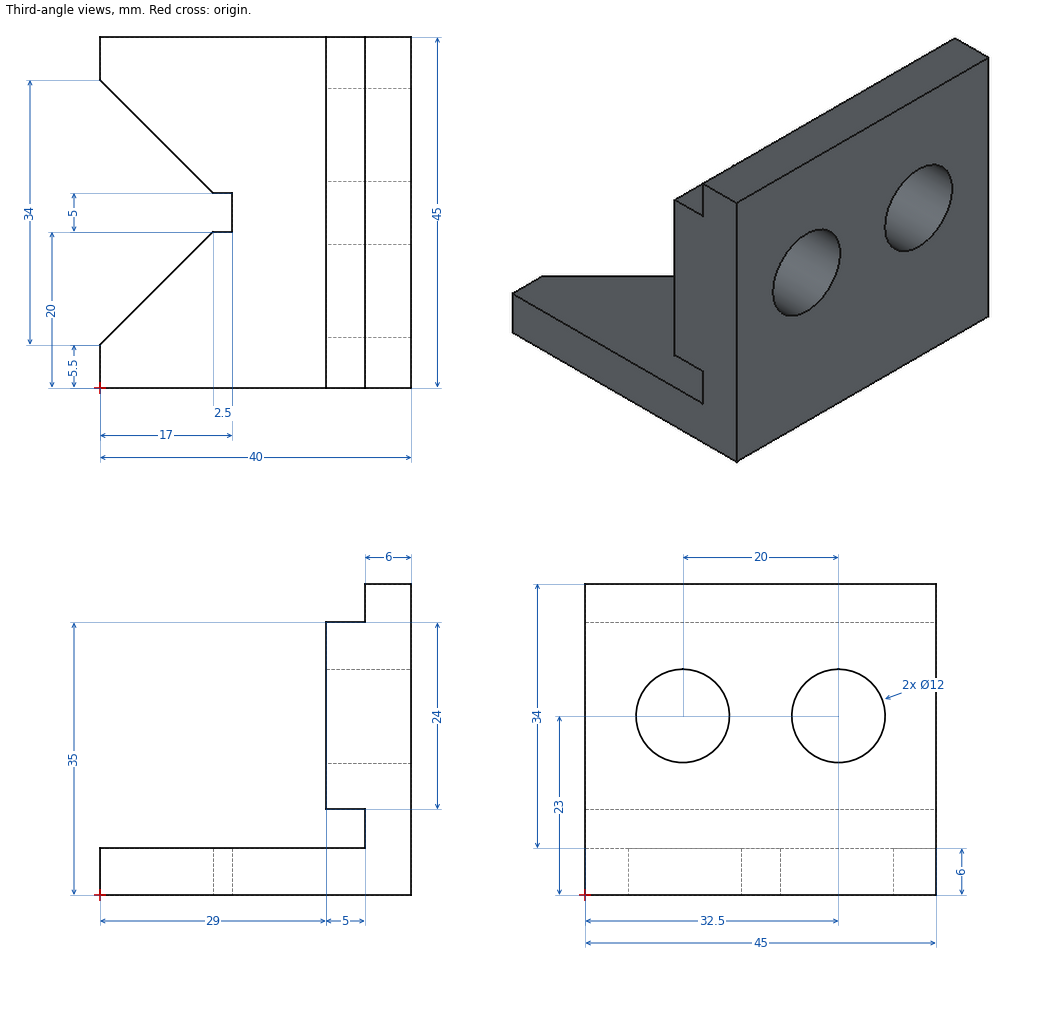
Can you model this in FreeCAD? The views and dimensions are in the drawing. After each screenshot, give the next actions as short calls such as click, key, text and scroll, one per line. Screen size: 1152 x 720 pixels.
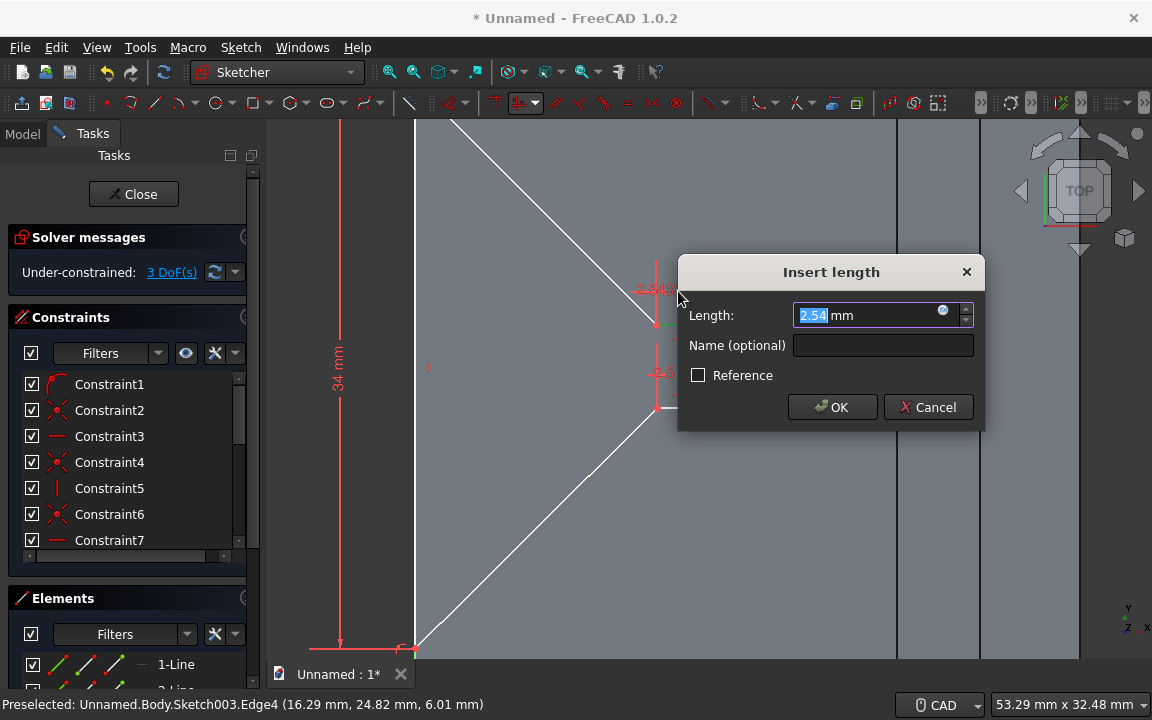
text(2.5)
key(Return)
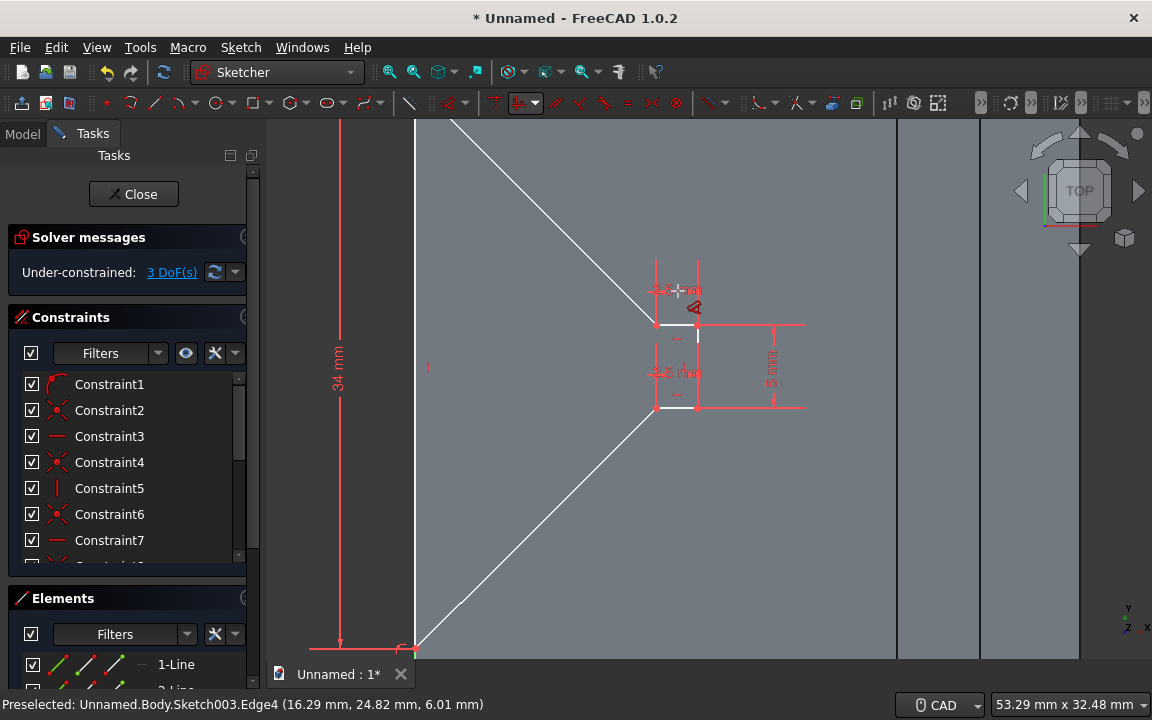
click(656, 408)
click(381, 520)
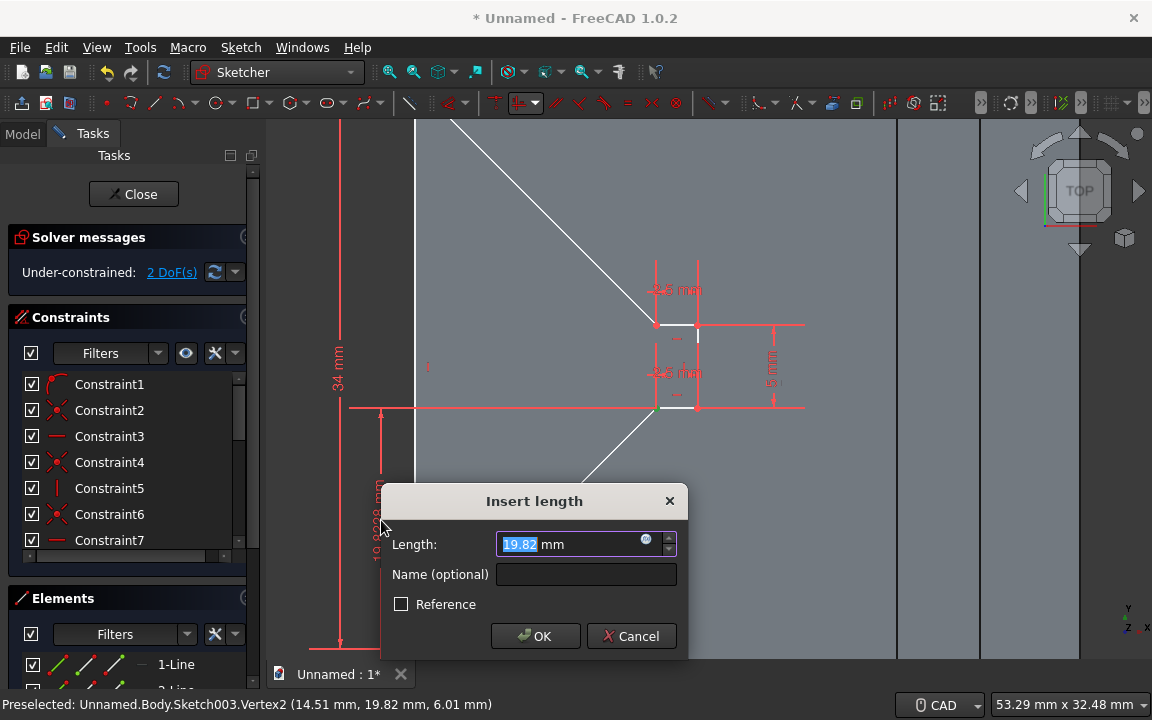
text(20)
key(Return)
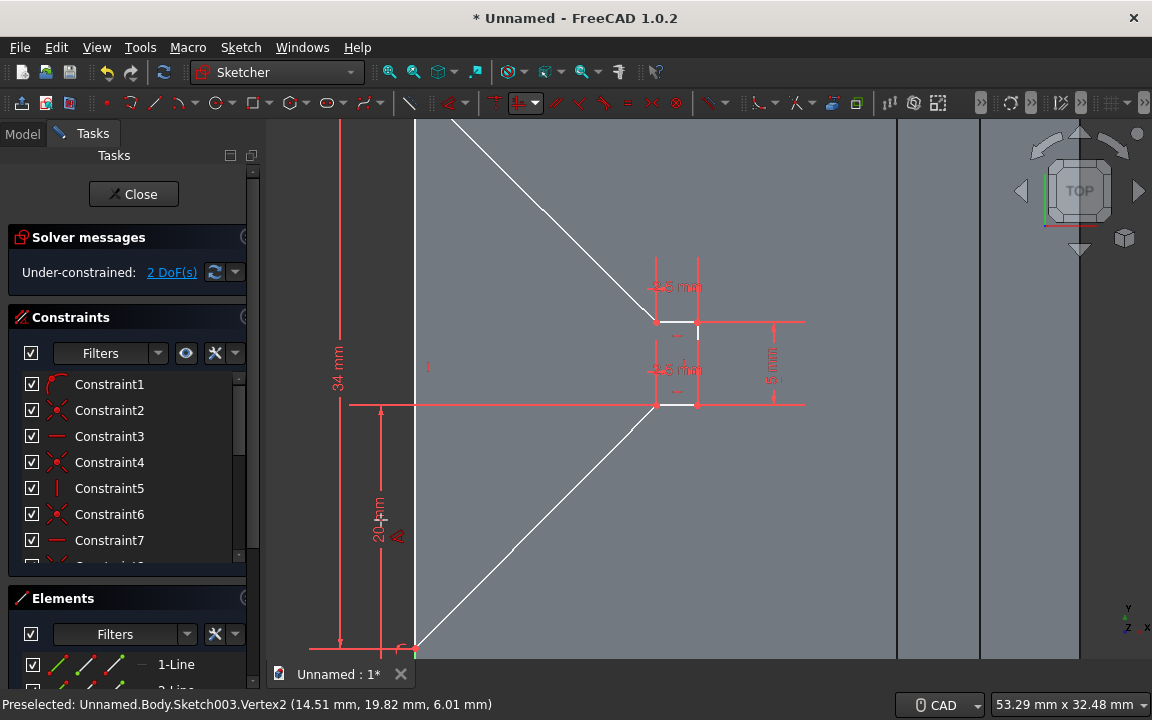
click(698, 405)
click(557, 371)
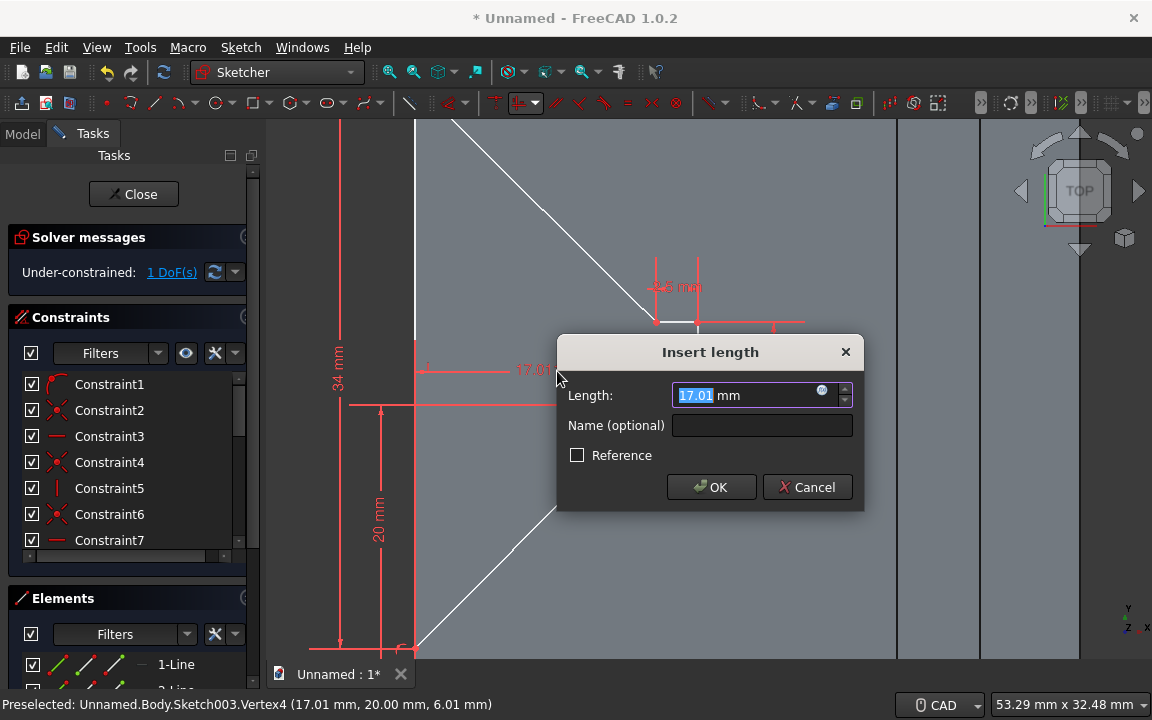
text(17)
key(Return)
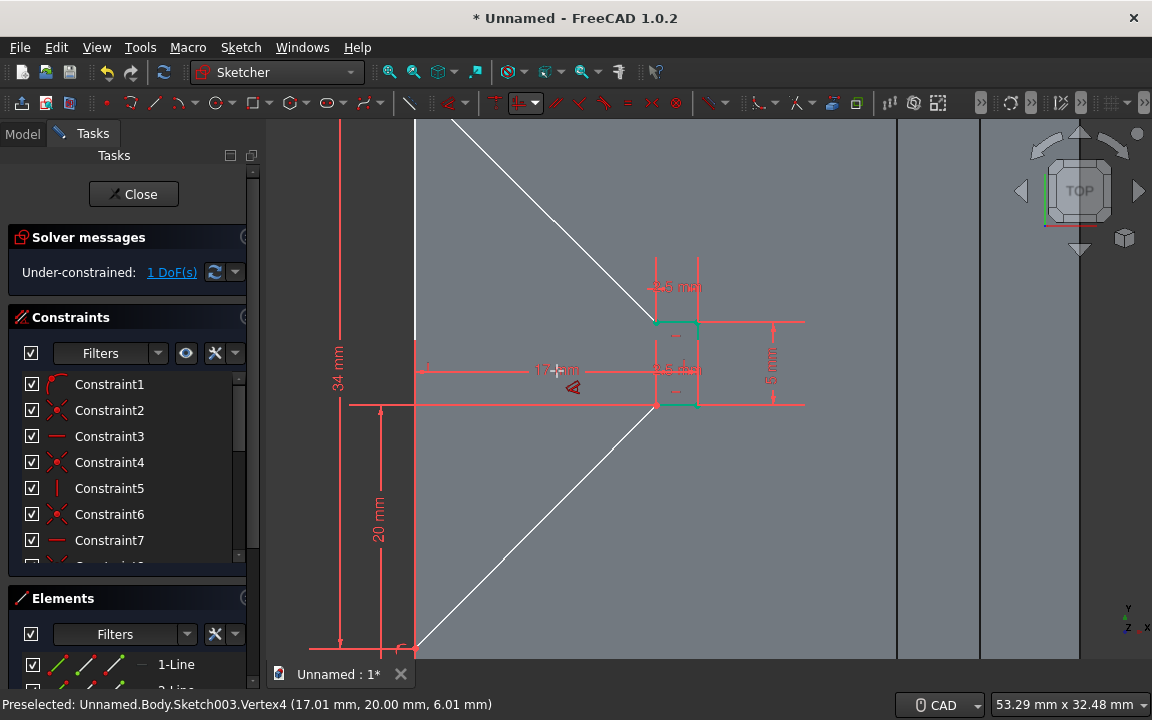
scroll(743, 364, down, 3)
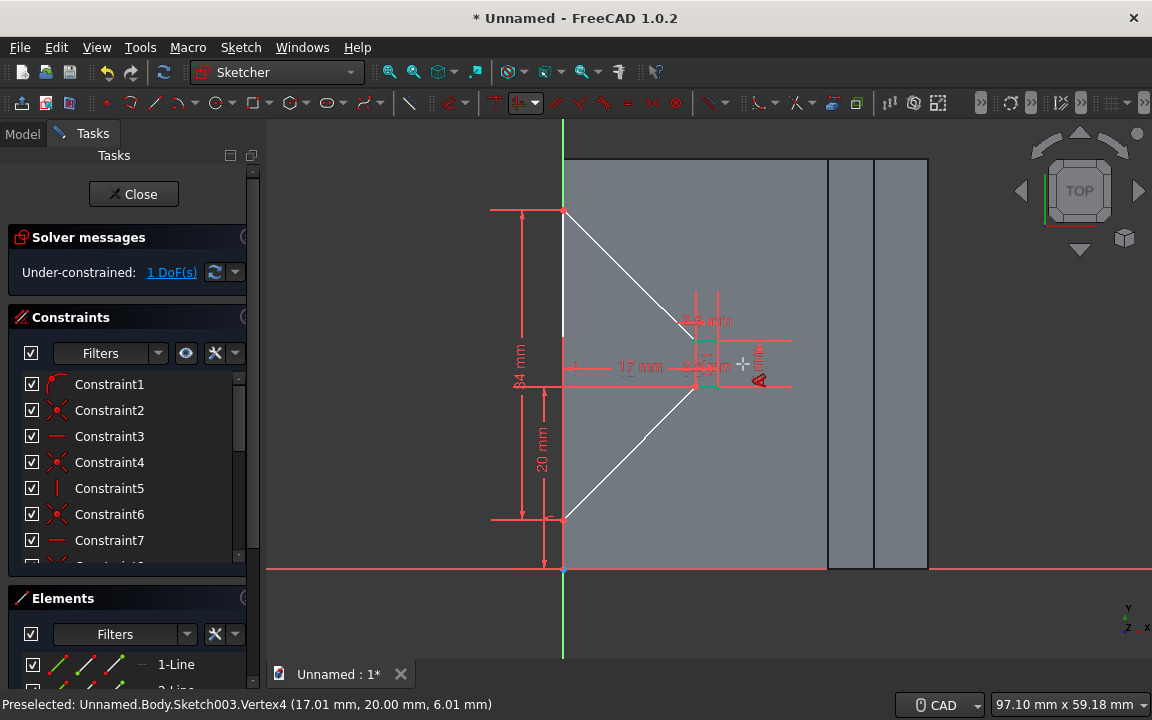
click(563, 520)
click(529, 545)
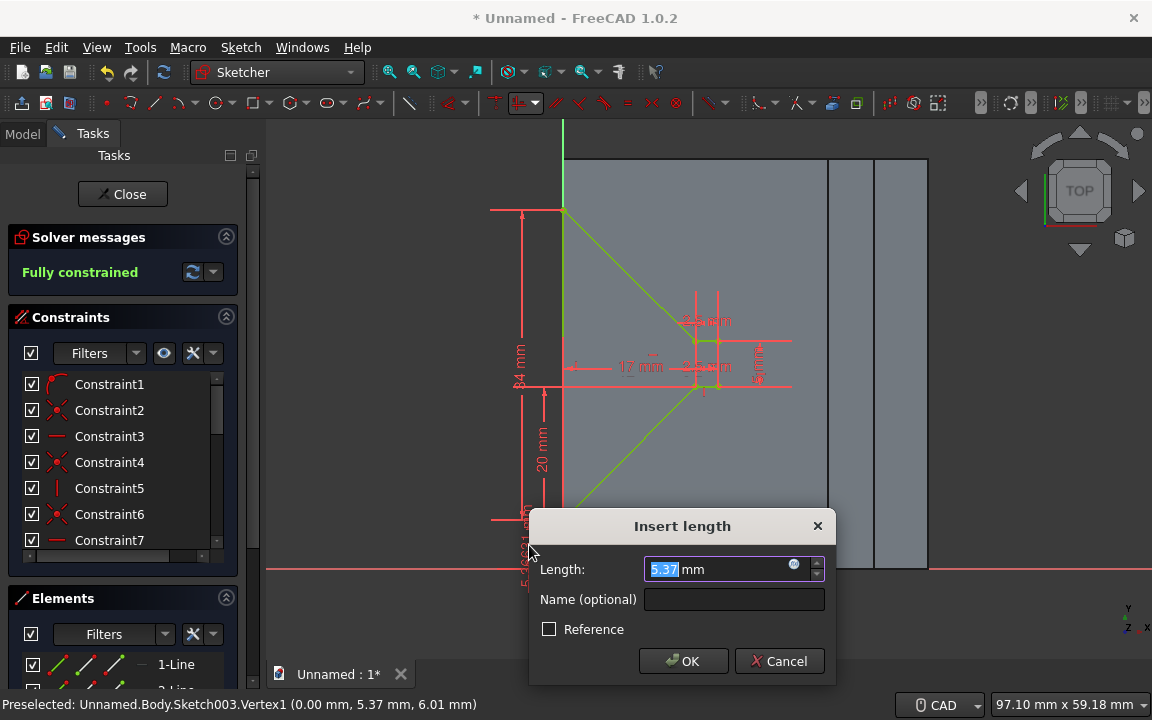
text(5.5)
key(Return)
key(Escape)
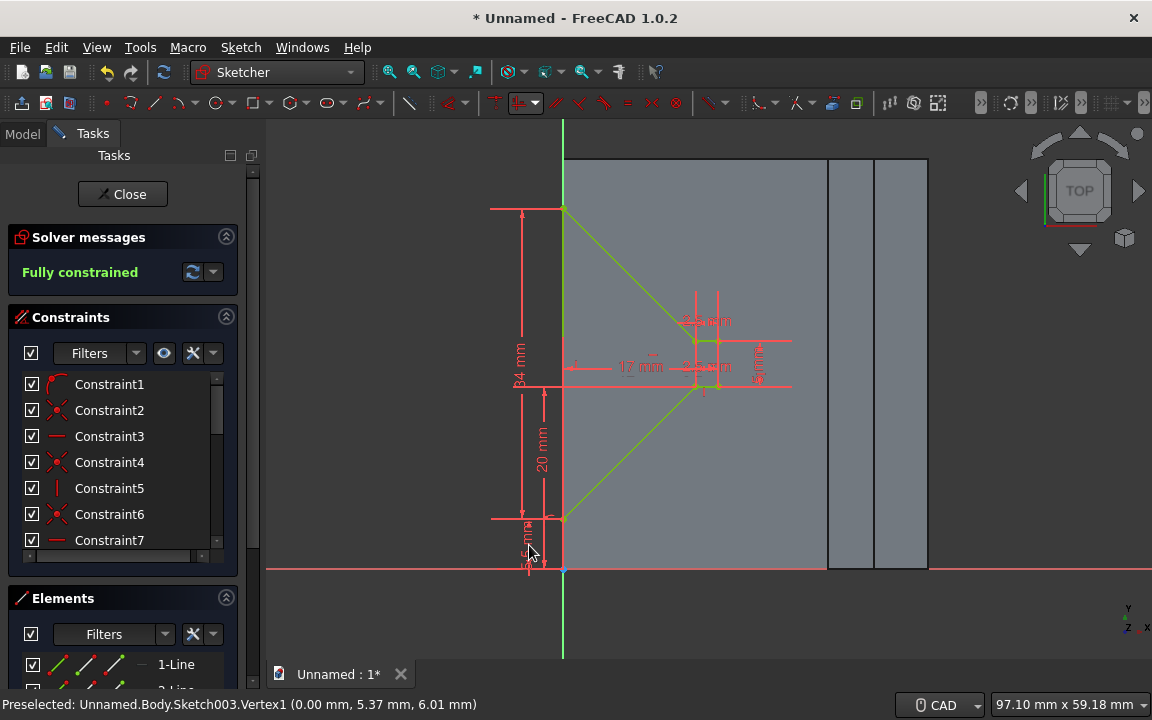
click(123, 194)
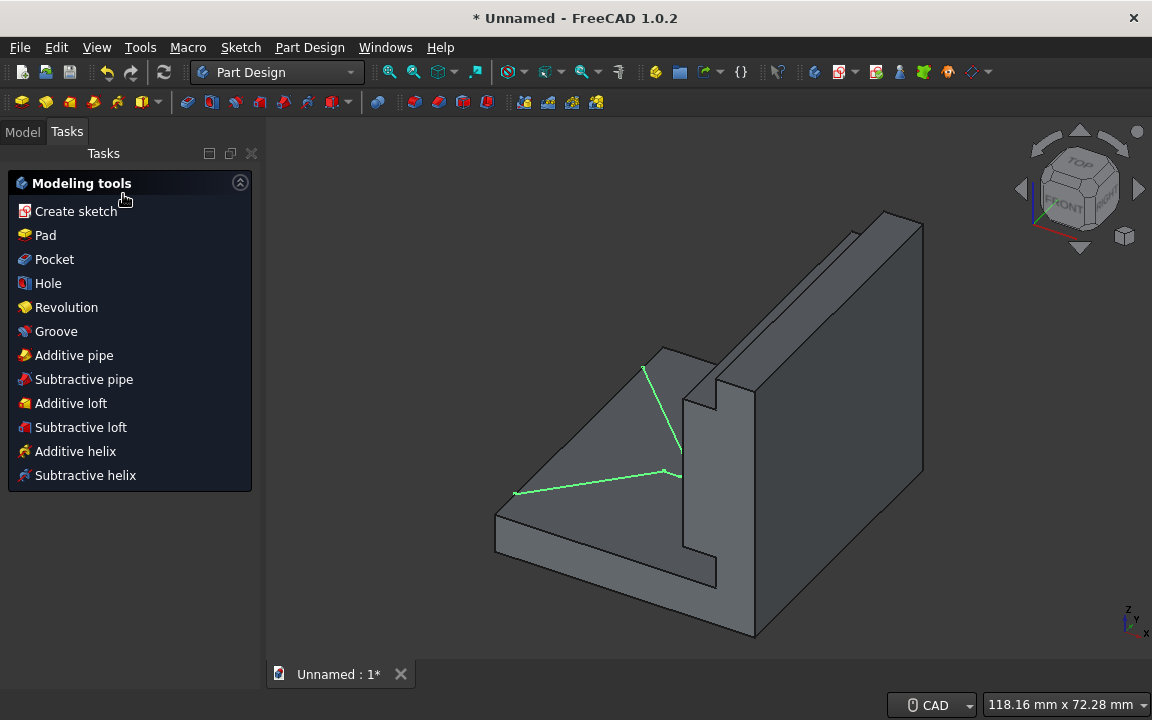
click(188, 102)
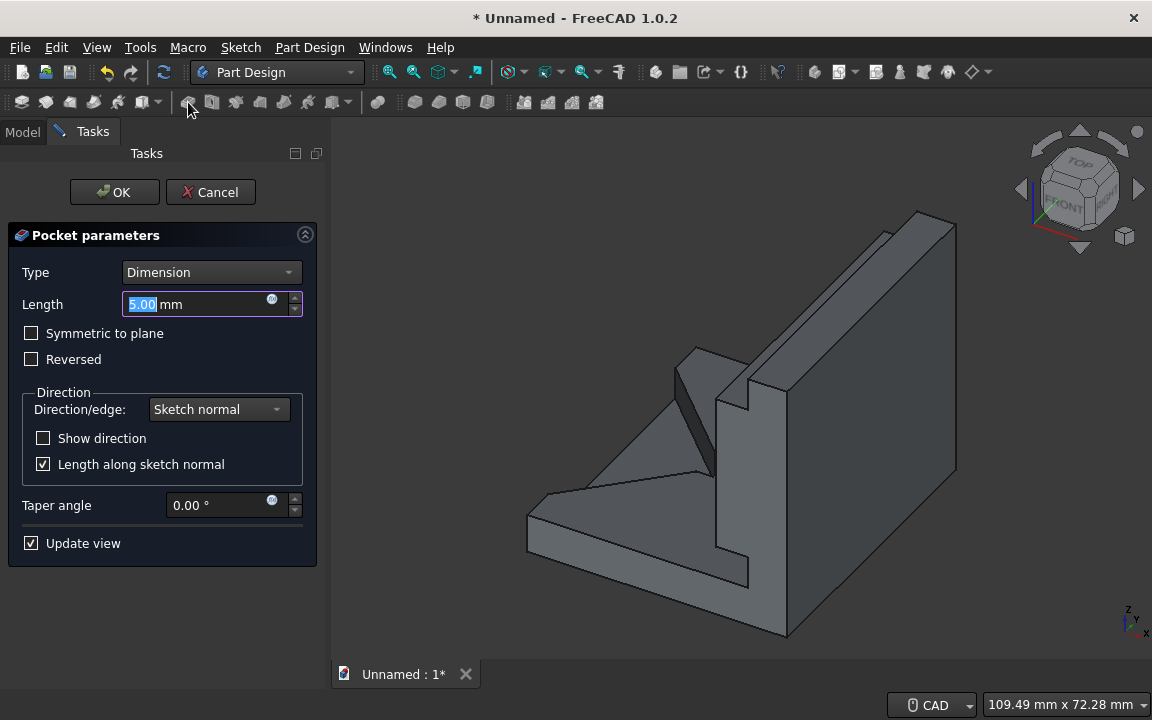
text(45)
key(Tab)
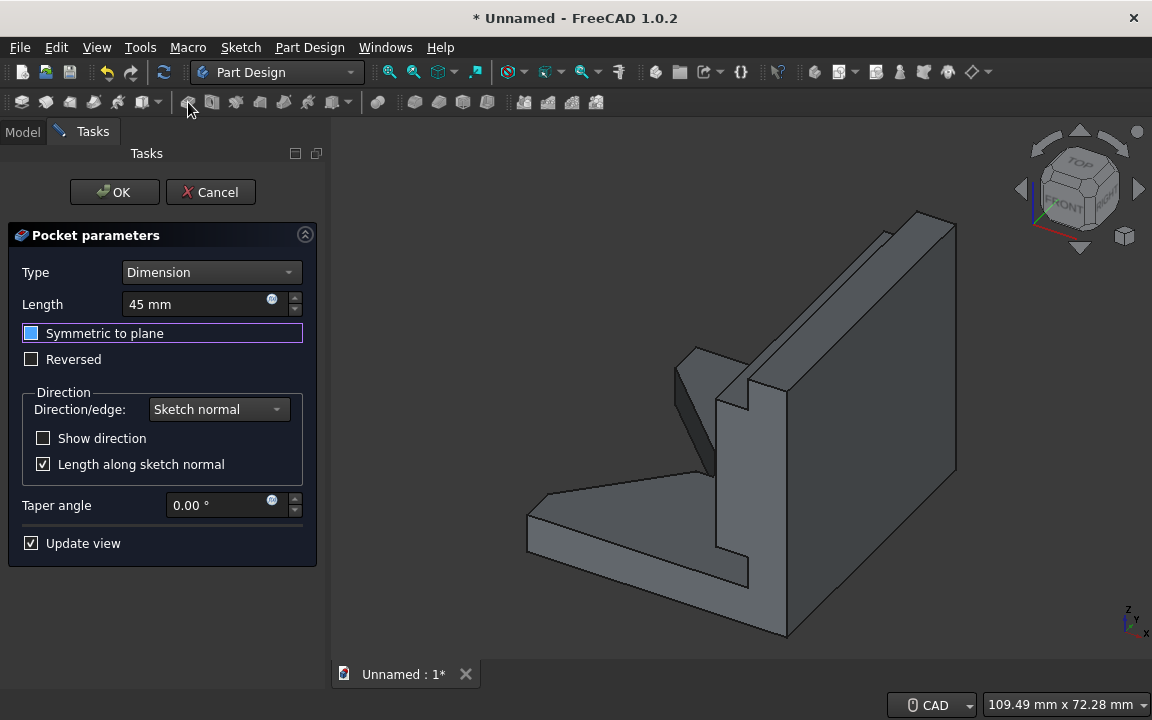
click(115, 192)